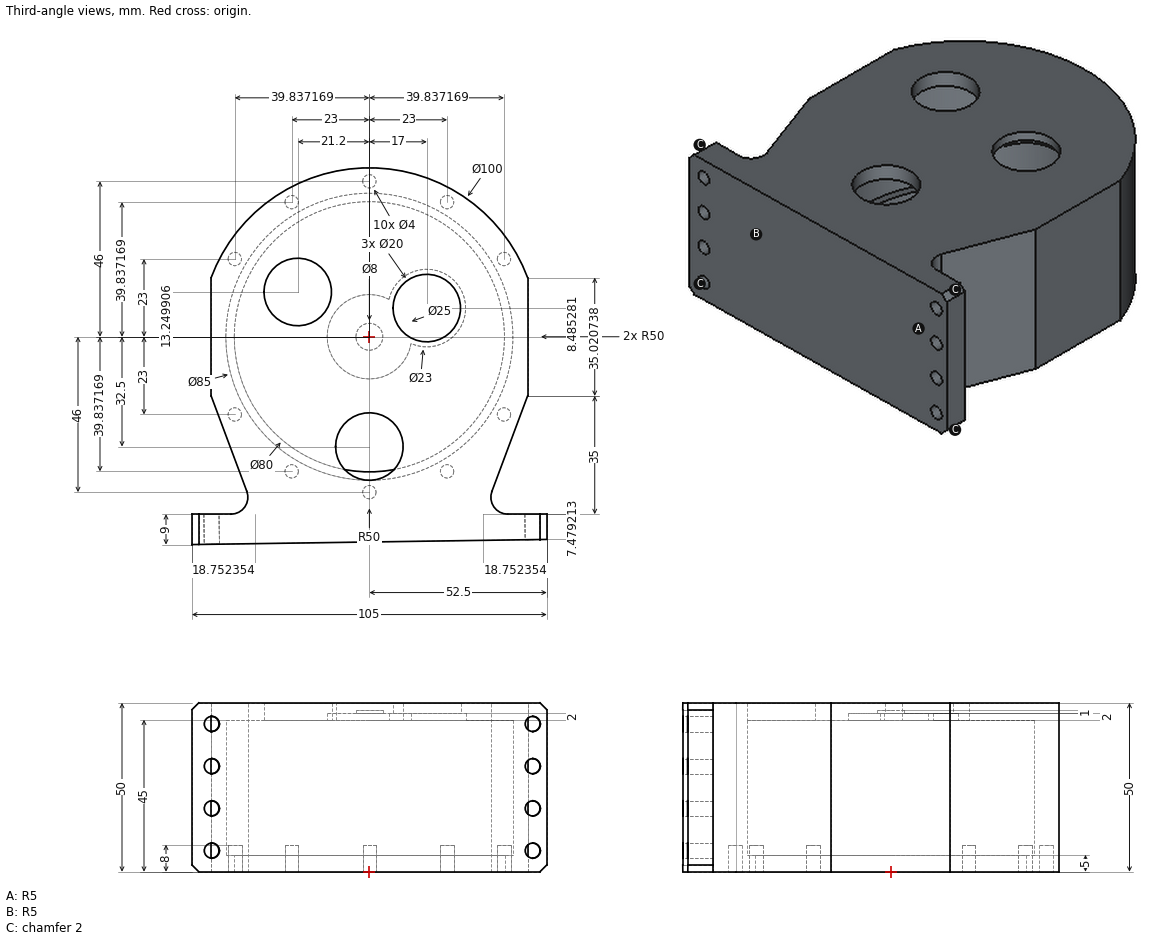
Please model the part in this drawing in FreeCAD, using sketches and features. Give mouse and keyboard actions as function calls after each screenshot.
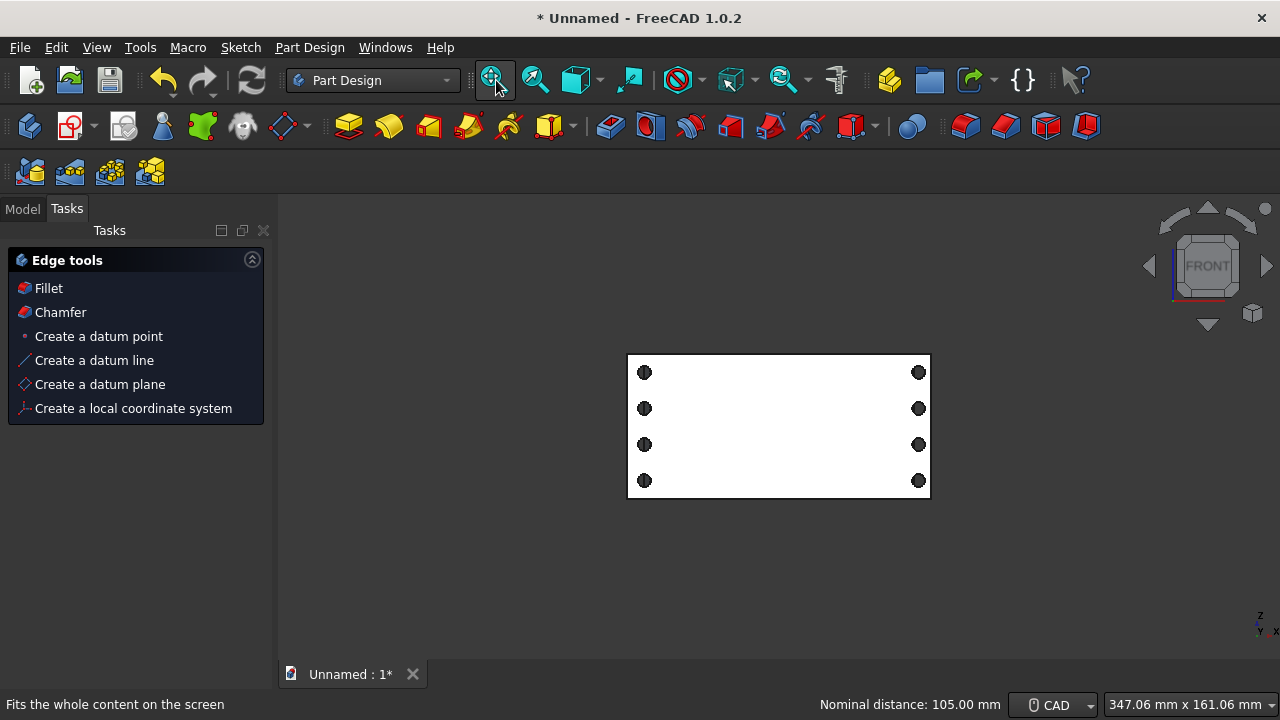
scroll(931, 498, up, 4)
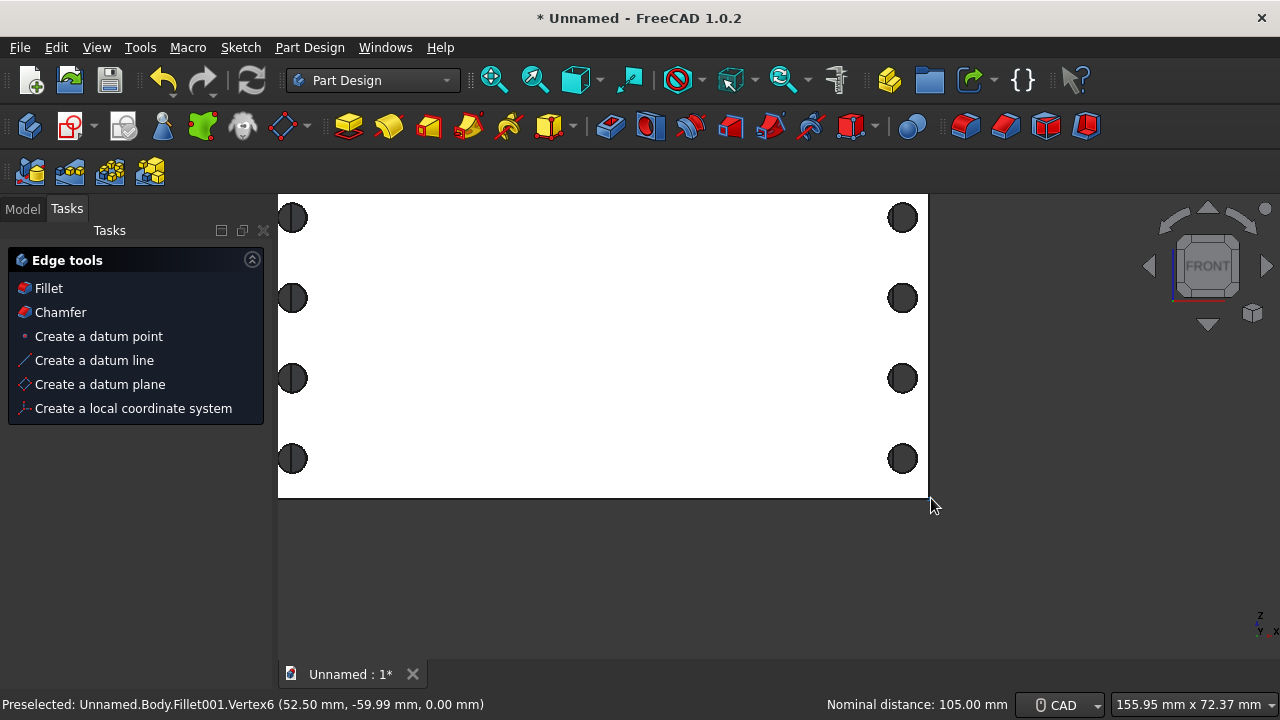
key(v)
key(f)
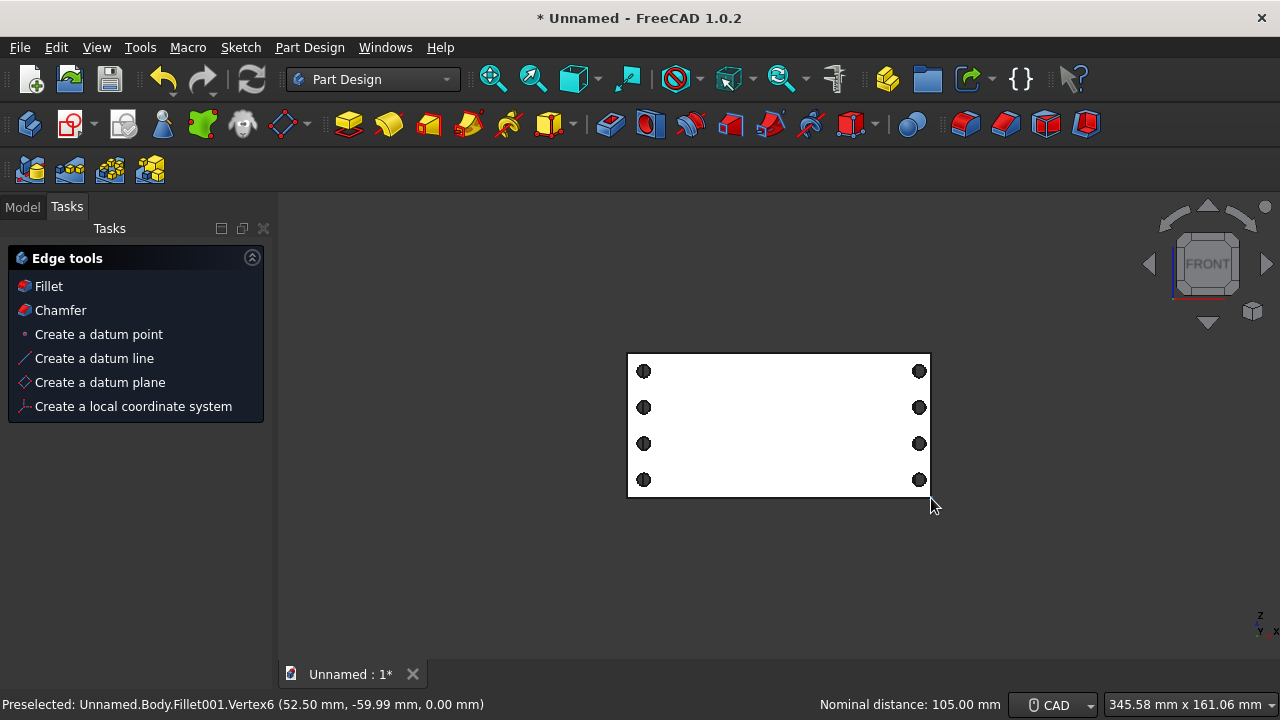
key(3)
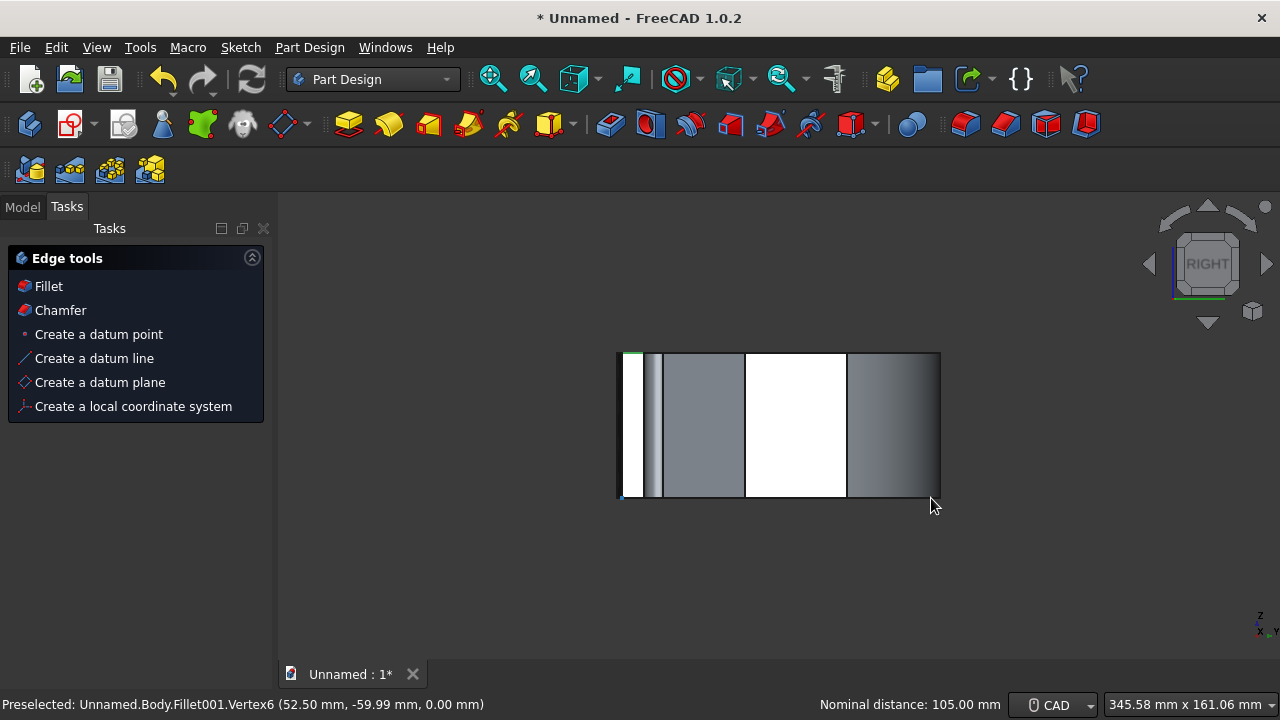
click(494, 80)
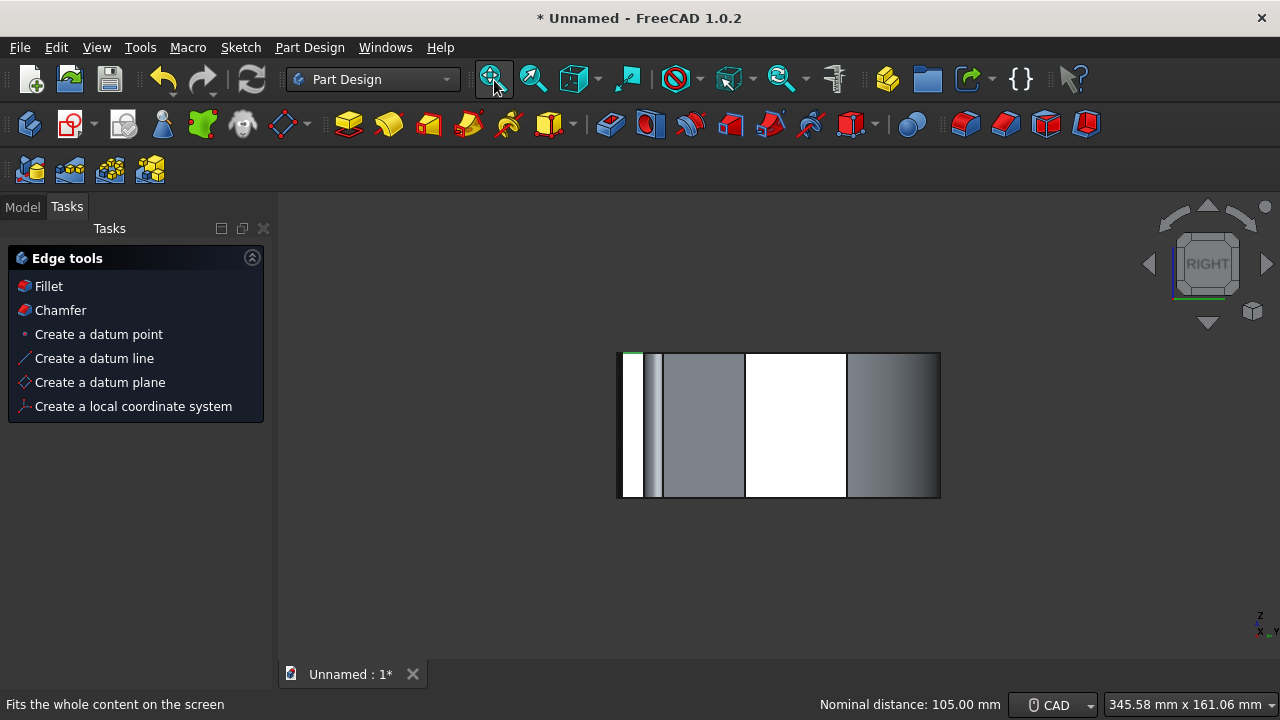
click(633, 497, ctrl)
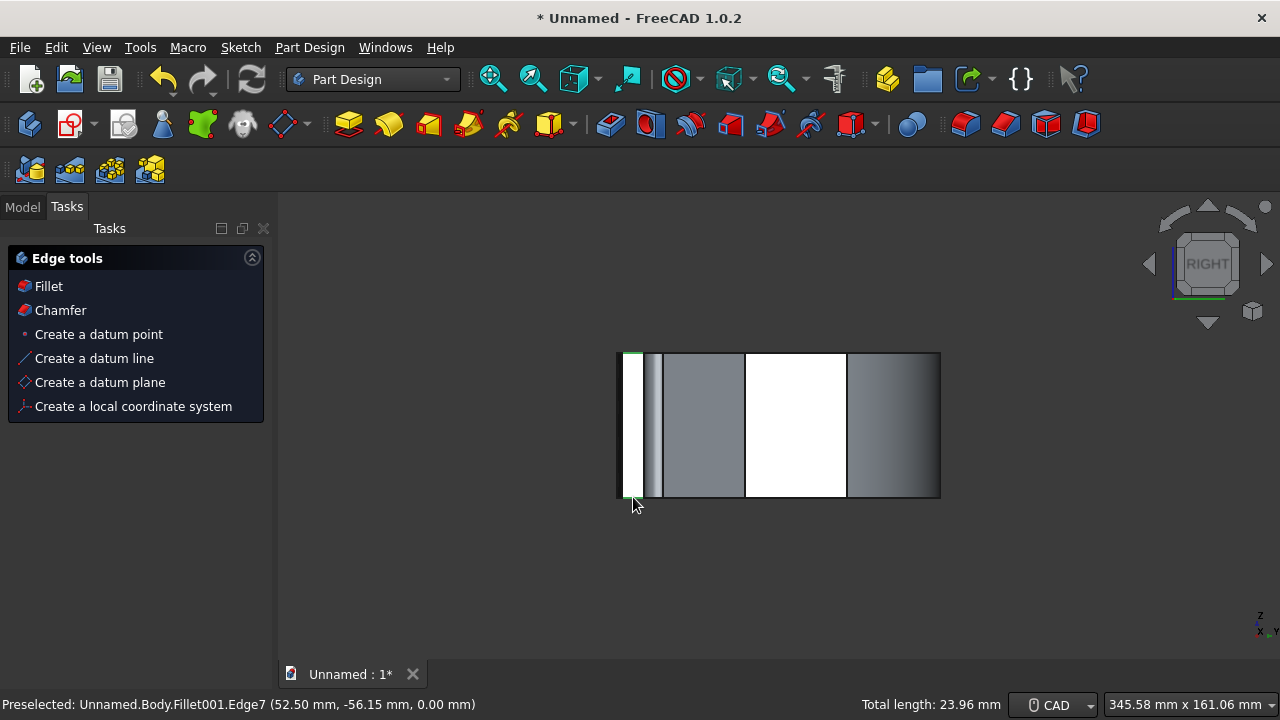
key(5)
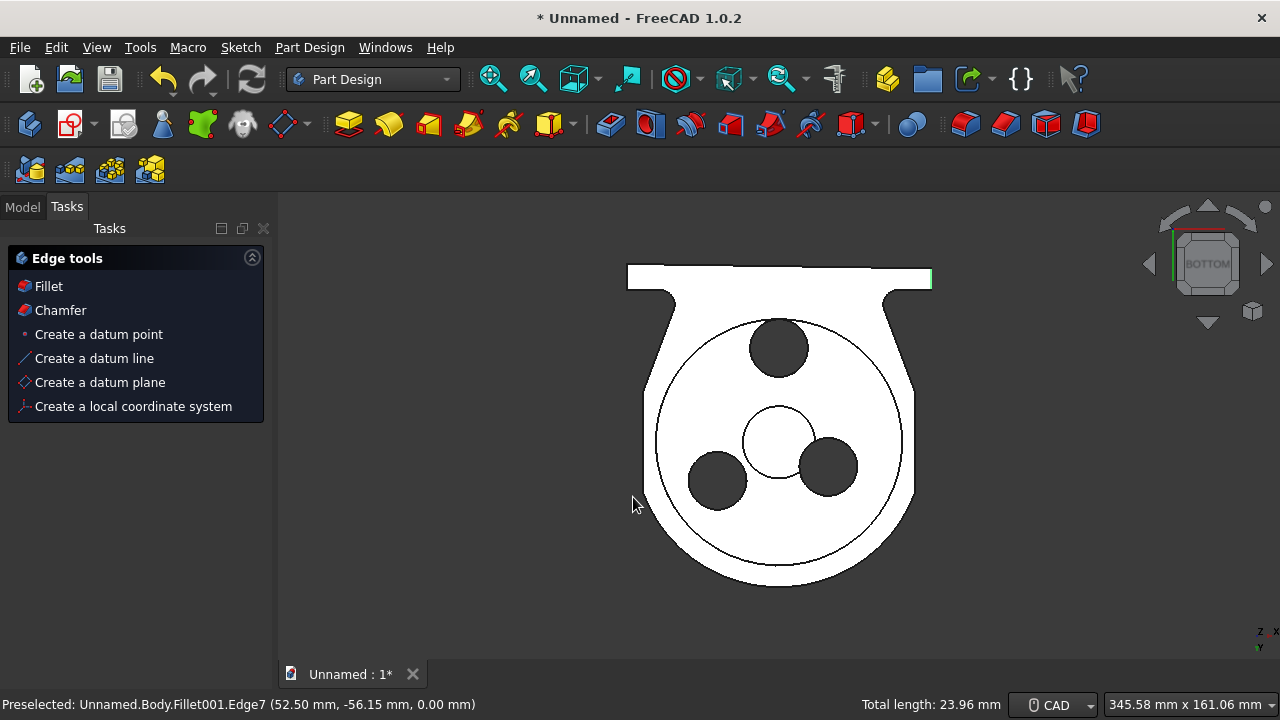
click(627, 276, ctrl)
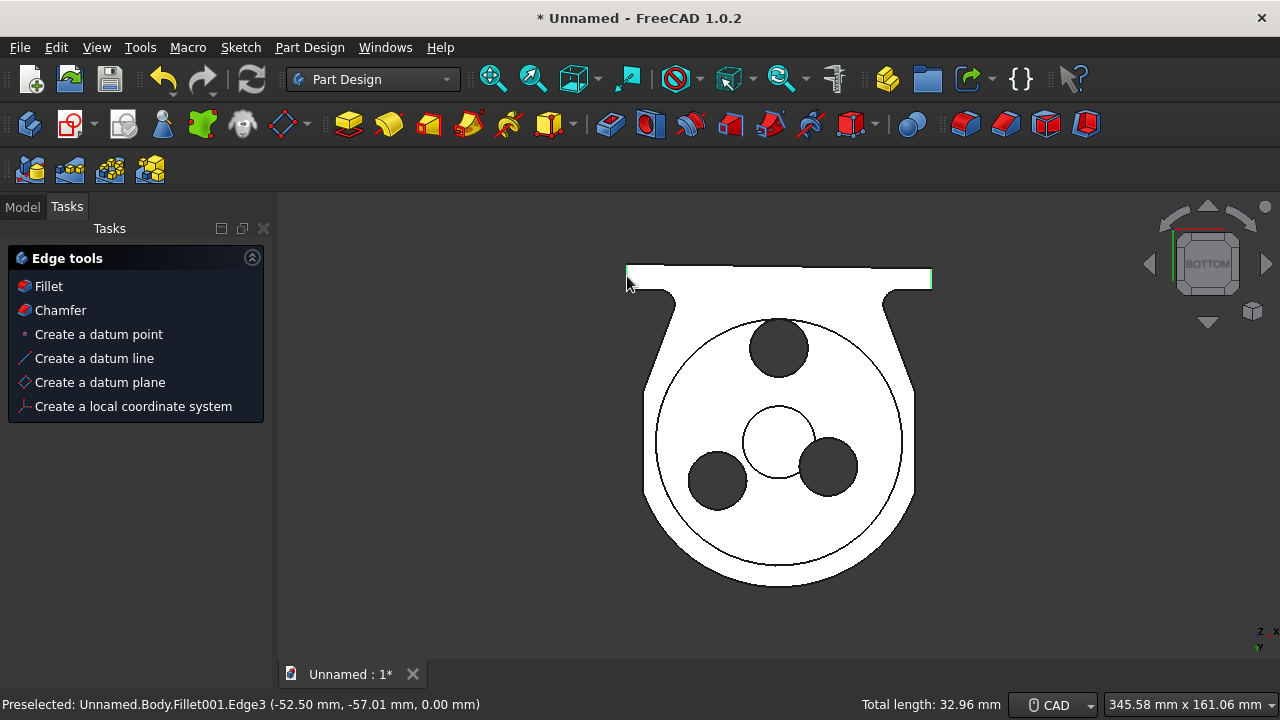
click(1006, 124)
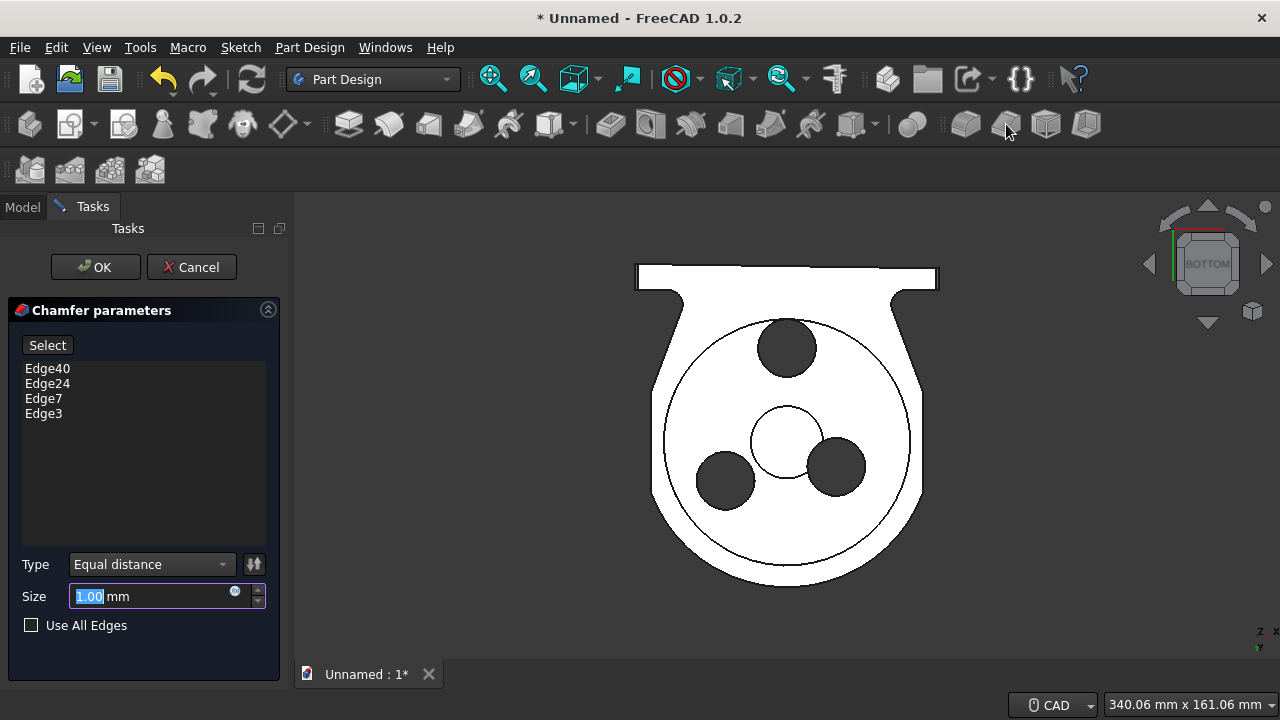
text(2)
key(Tab)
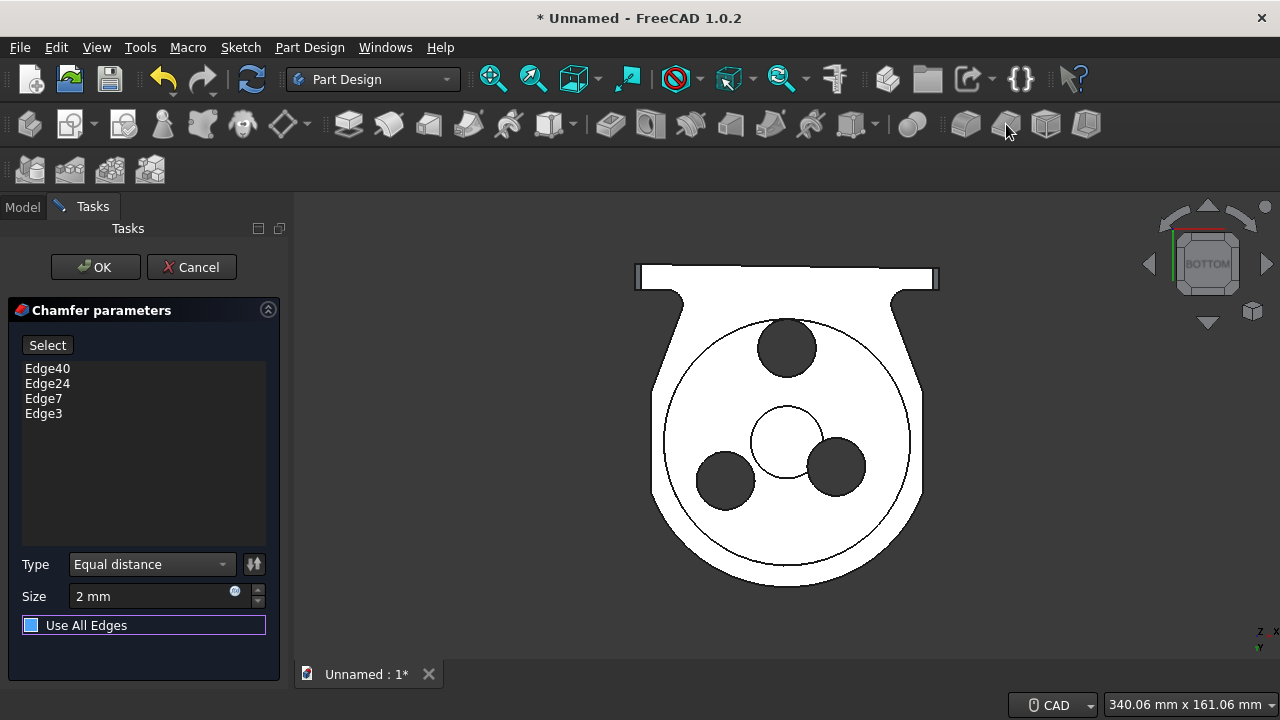
click(96, 267)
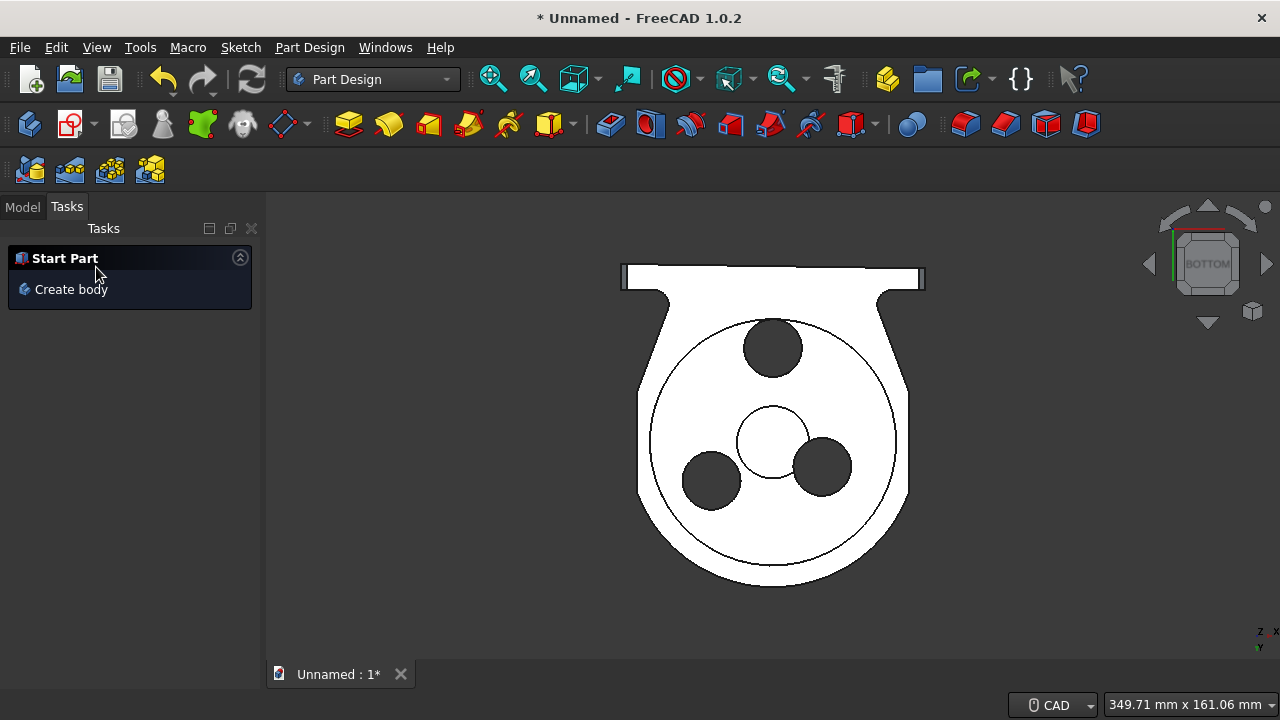
click(773, 441)